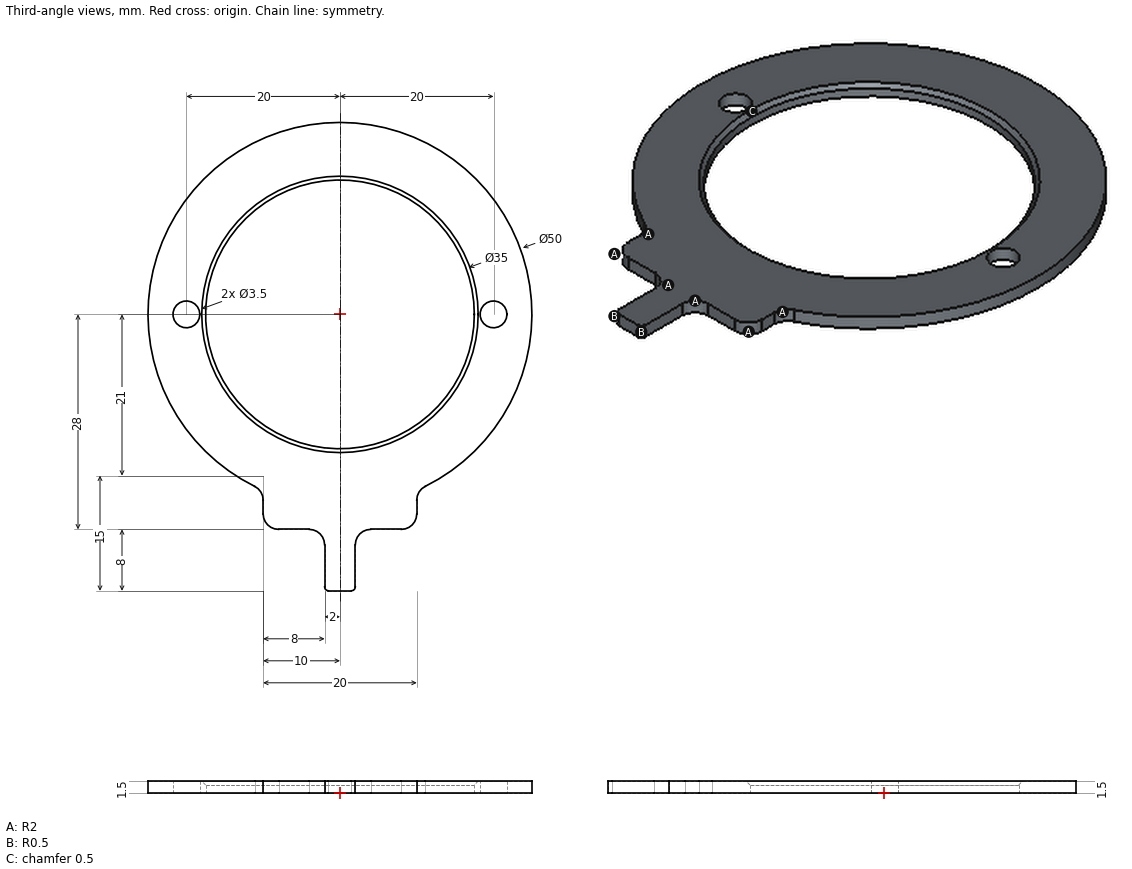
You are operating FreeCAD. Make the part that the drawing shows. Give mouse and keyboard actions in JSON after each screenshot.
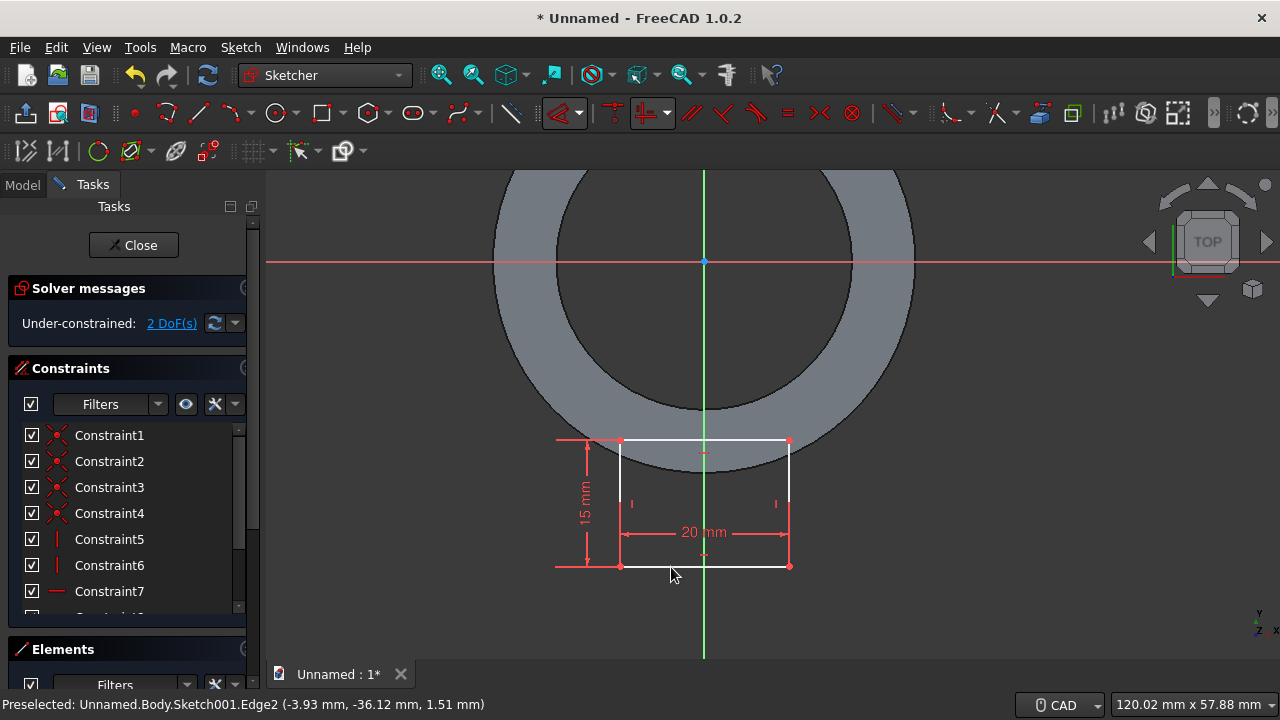
{"action": "left_click", "coordinate": [620, 440]}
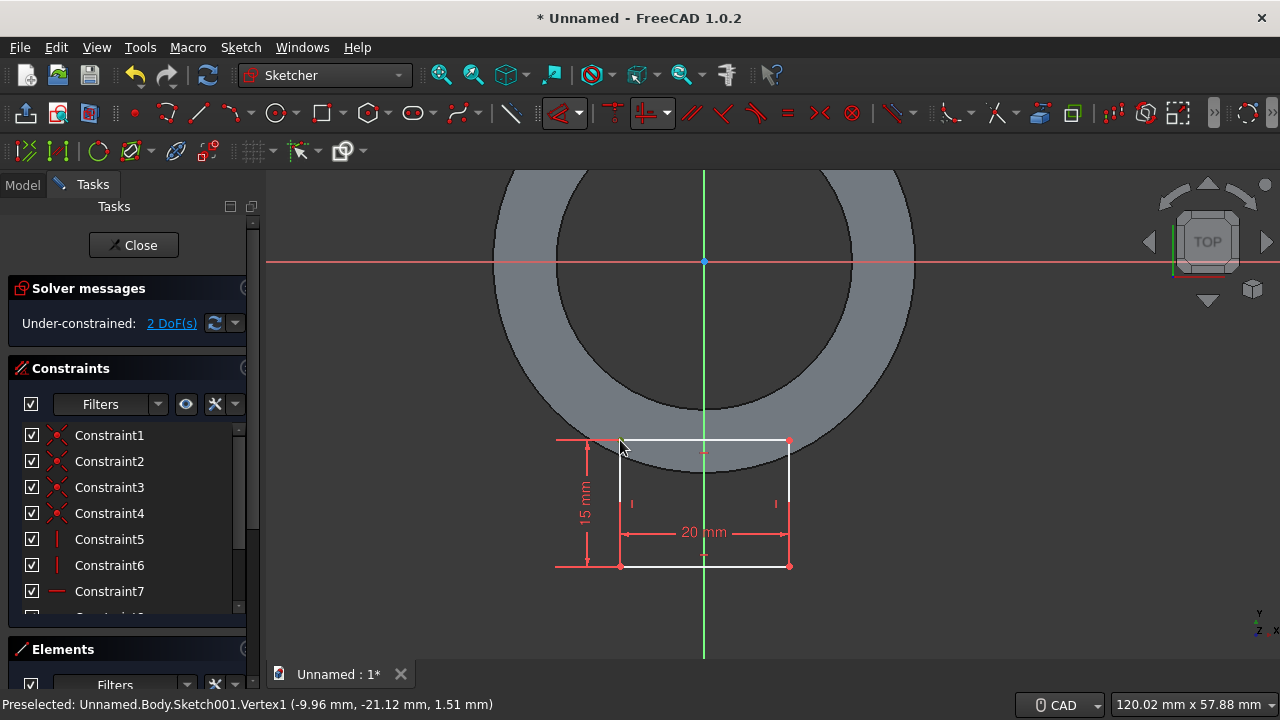
{"action": "left_click", "coordinate": [582, 114]}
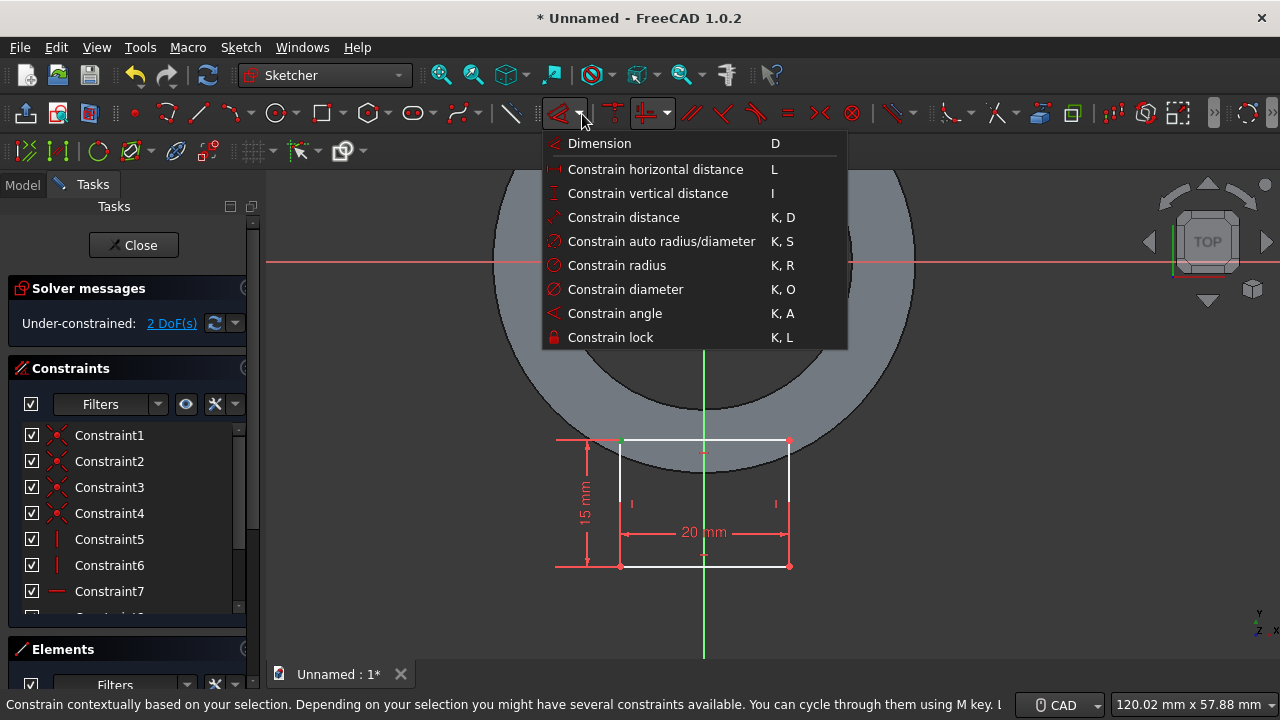
{"action": "left_click", "coordinate": [695, 169]}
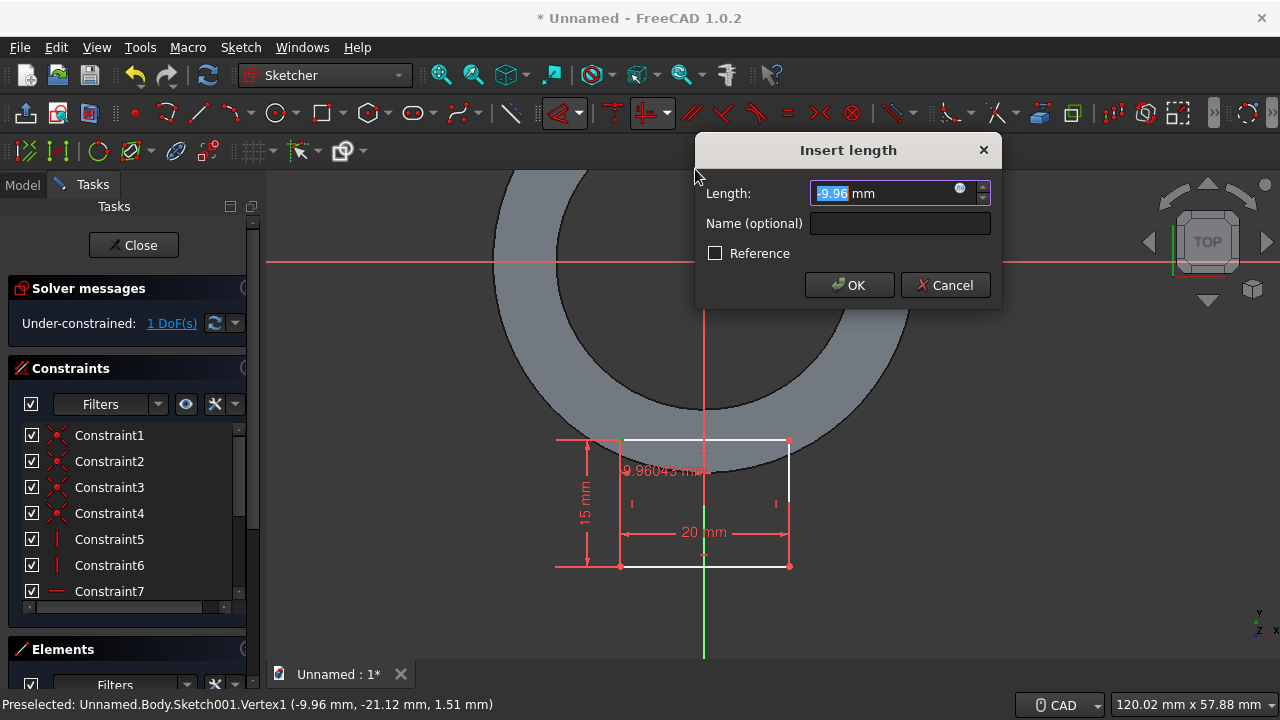
{"action": "type", "text": "-10"}
{"action": "key", "text": "Return"}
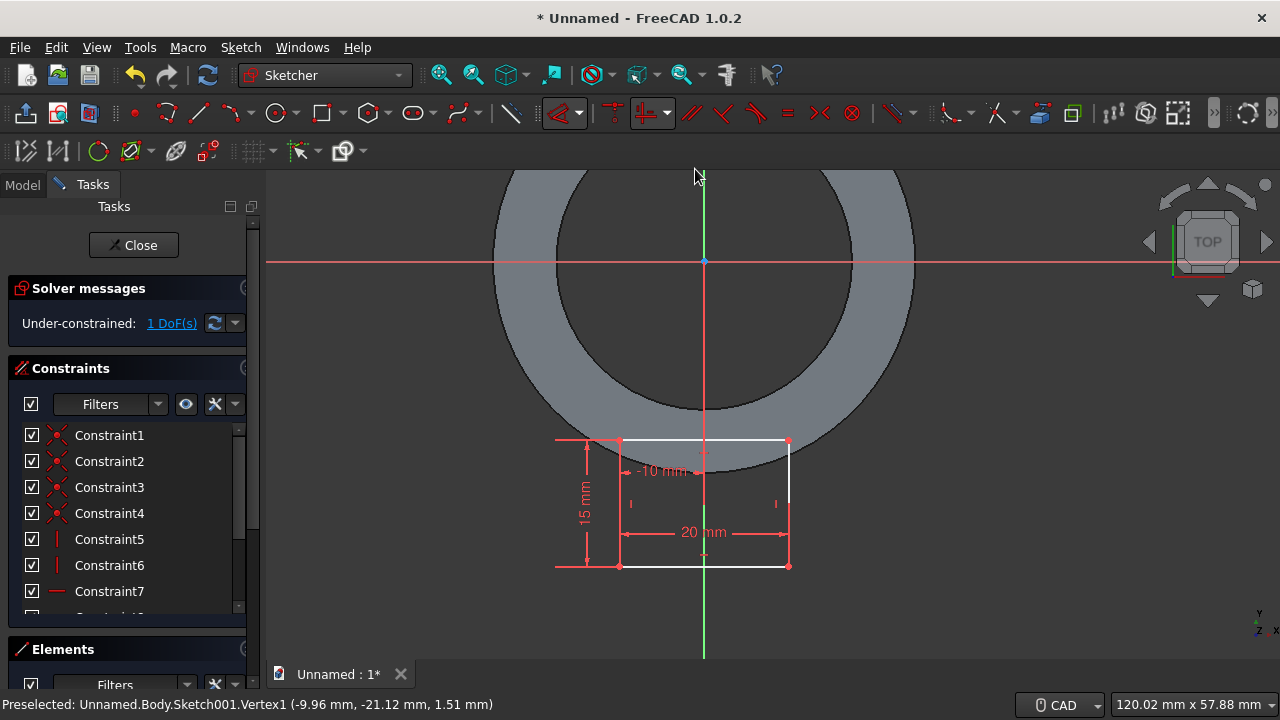
{"action": "left_click", "coordinate": [620, 440]}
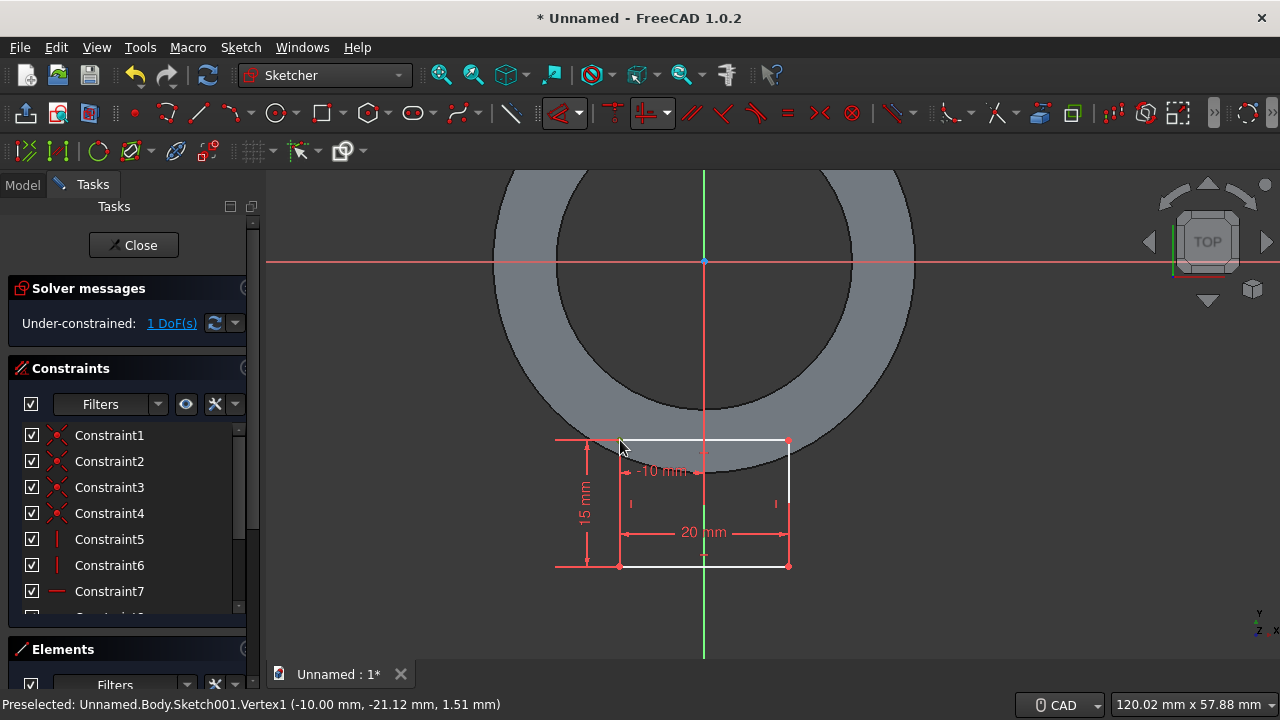
{"action": "left_click", "coordinate": [582, 114]}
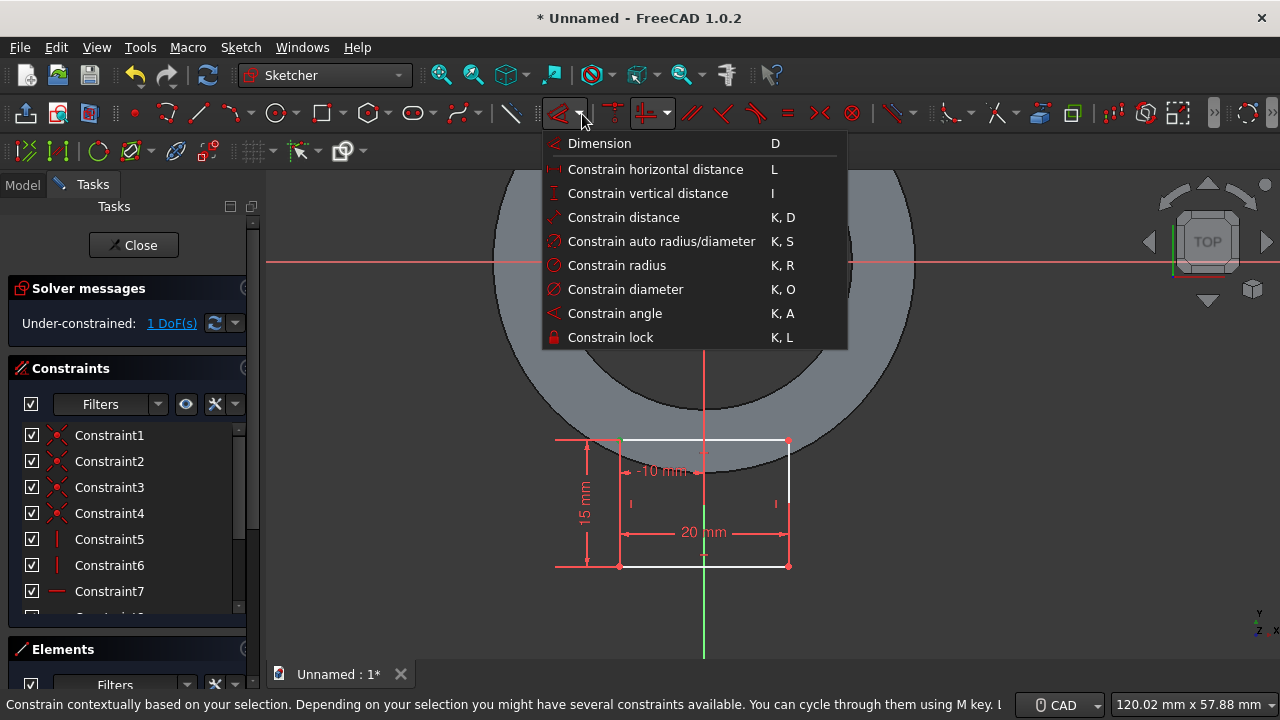
{"action": "left_click", "coordinate": [695, 193]}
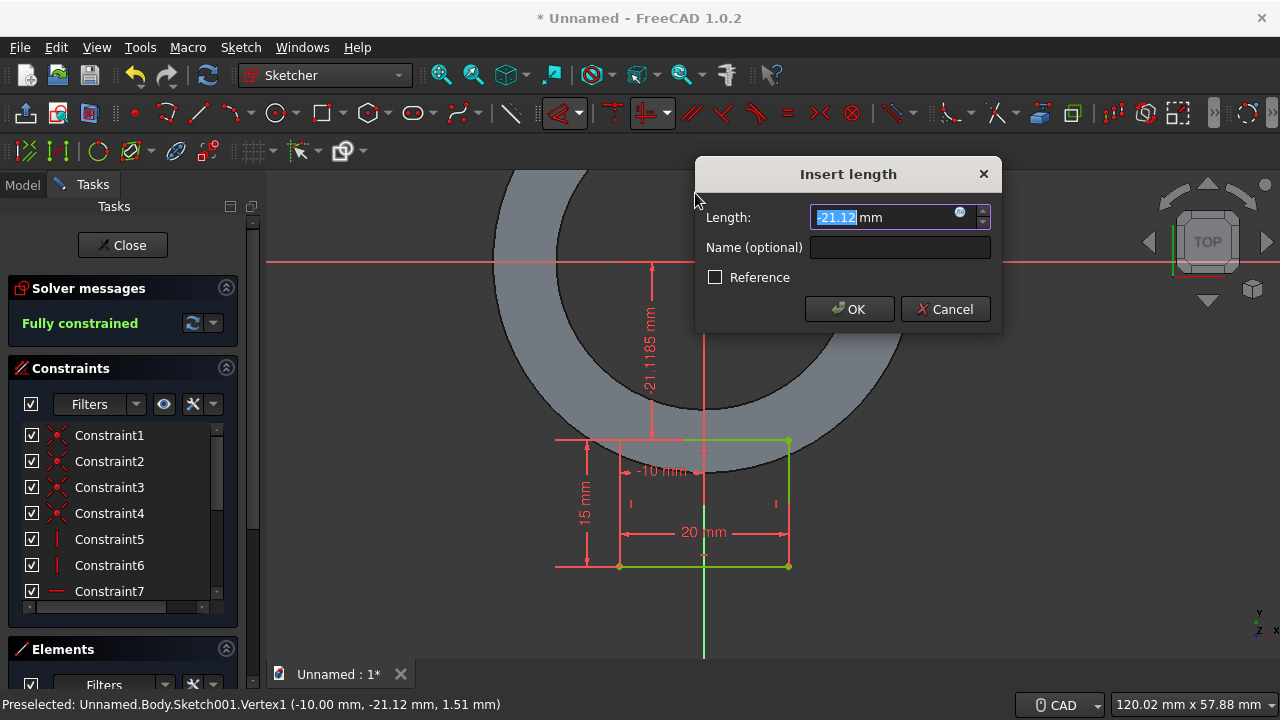
{"action": "type", "text": "-21"}
{"action": "key", "text": "Return"}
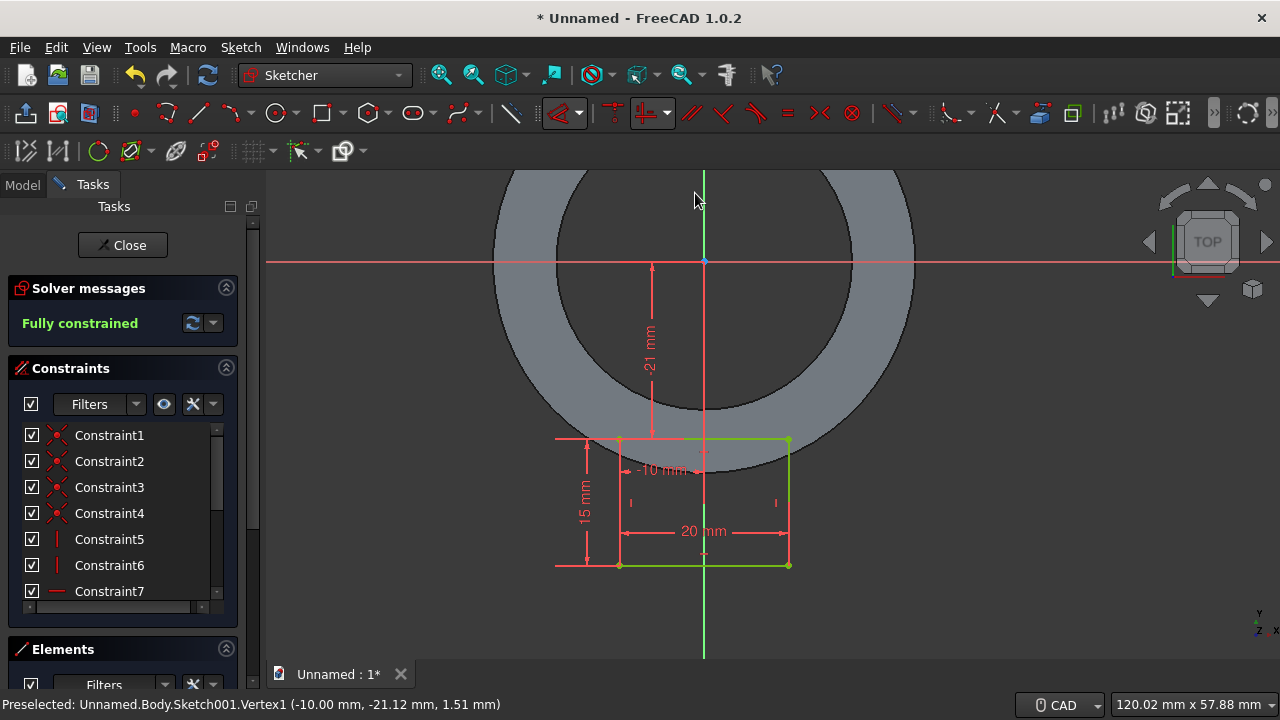
{"action": "left_click", "coordinate": [123, 245]}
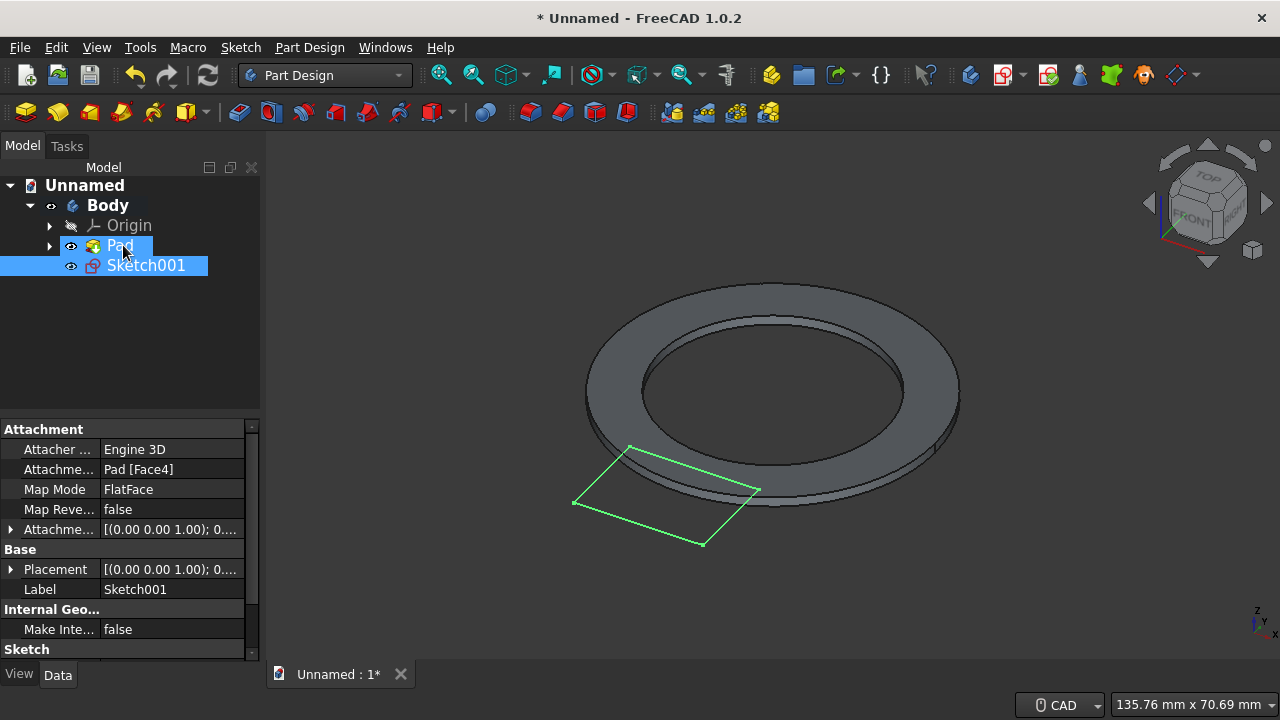
{"action": "left_click", "coordinate": [26, 112]}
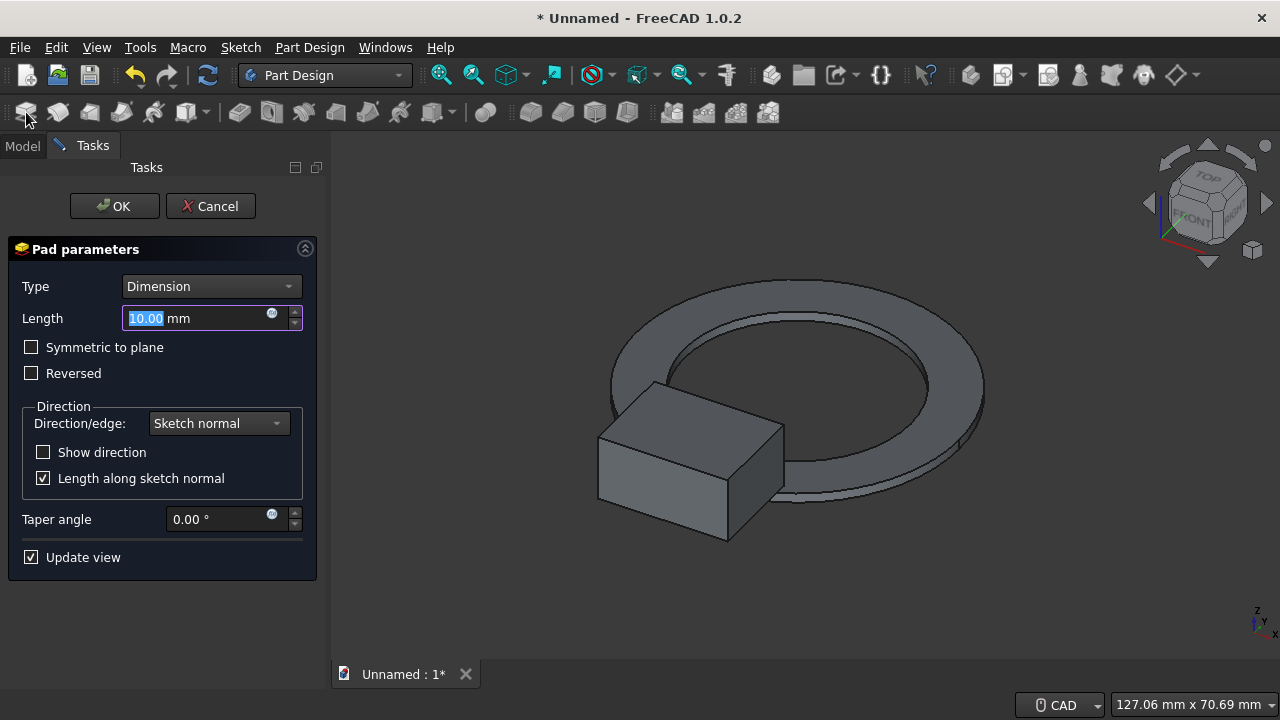
{"action": "type", "text": "1.5"}
{"action": "key", "text": "Tab"}